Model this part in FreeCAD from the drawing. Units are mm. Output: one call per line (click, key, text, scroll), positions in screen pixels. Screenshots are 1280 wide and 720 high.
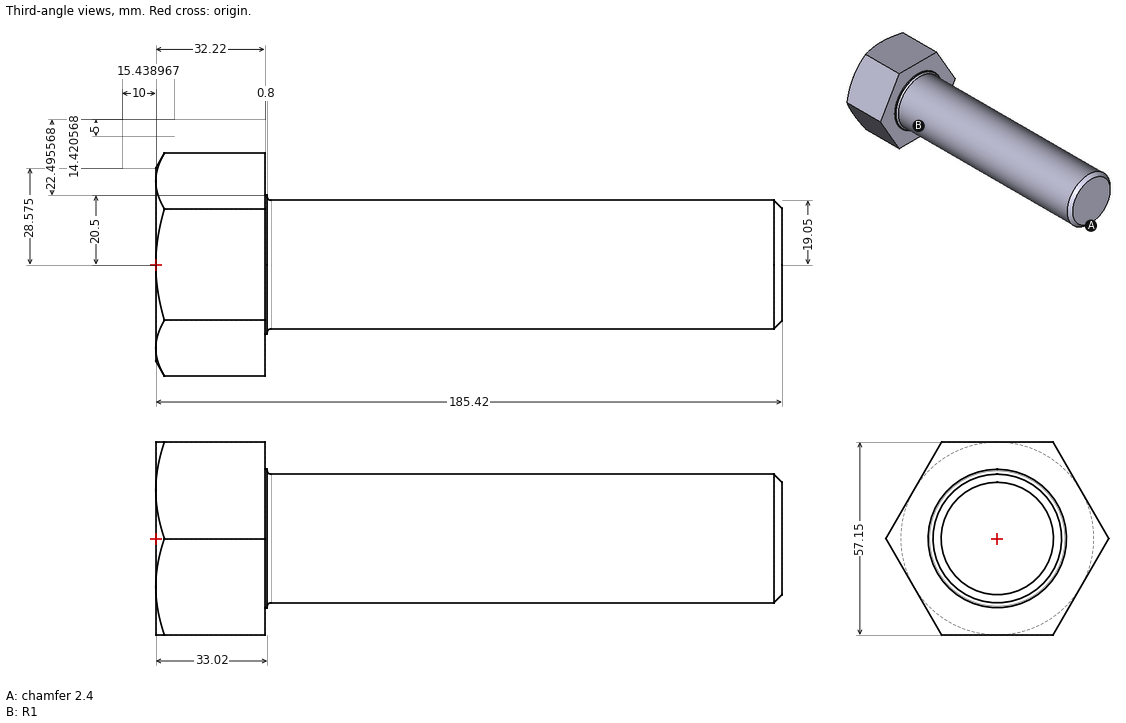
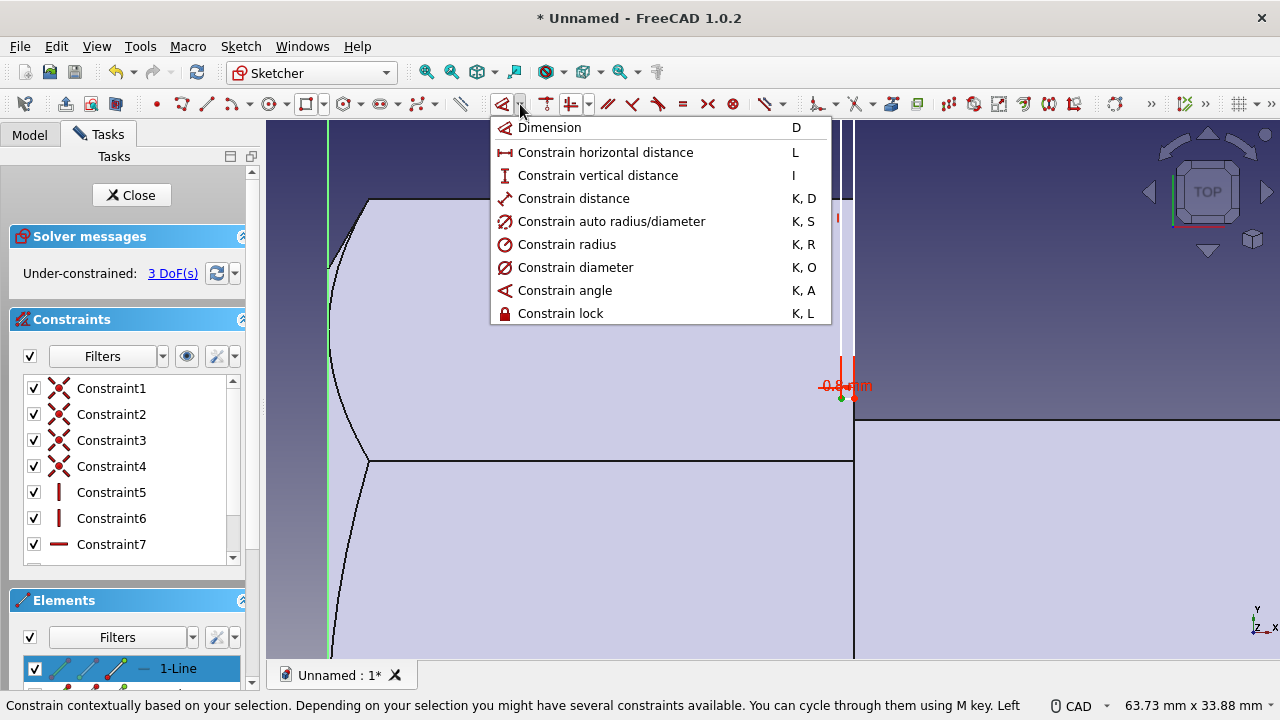
click(661, 176)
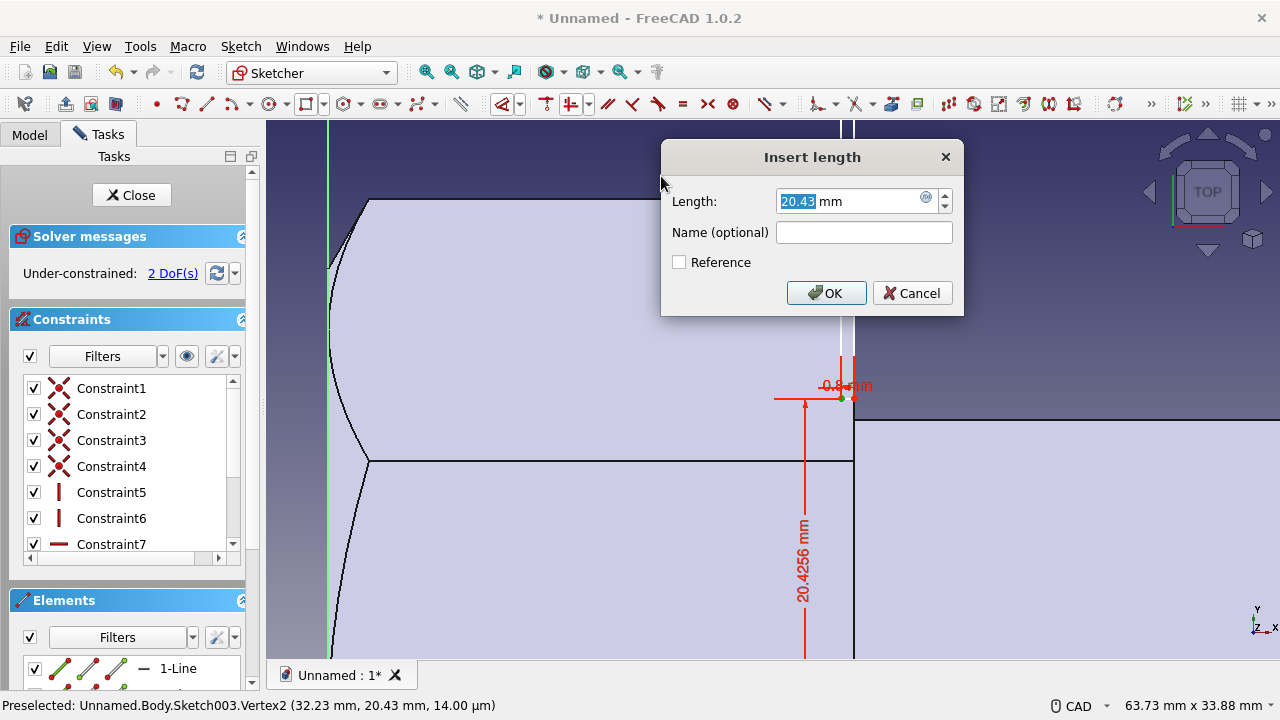
text(20.5)
key(Return)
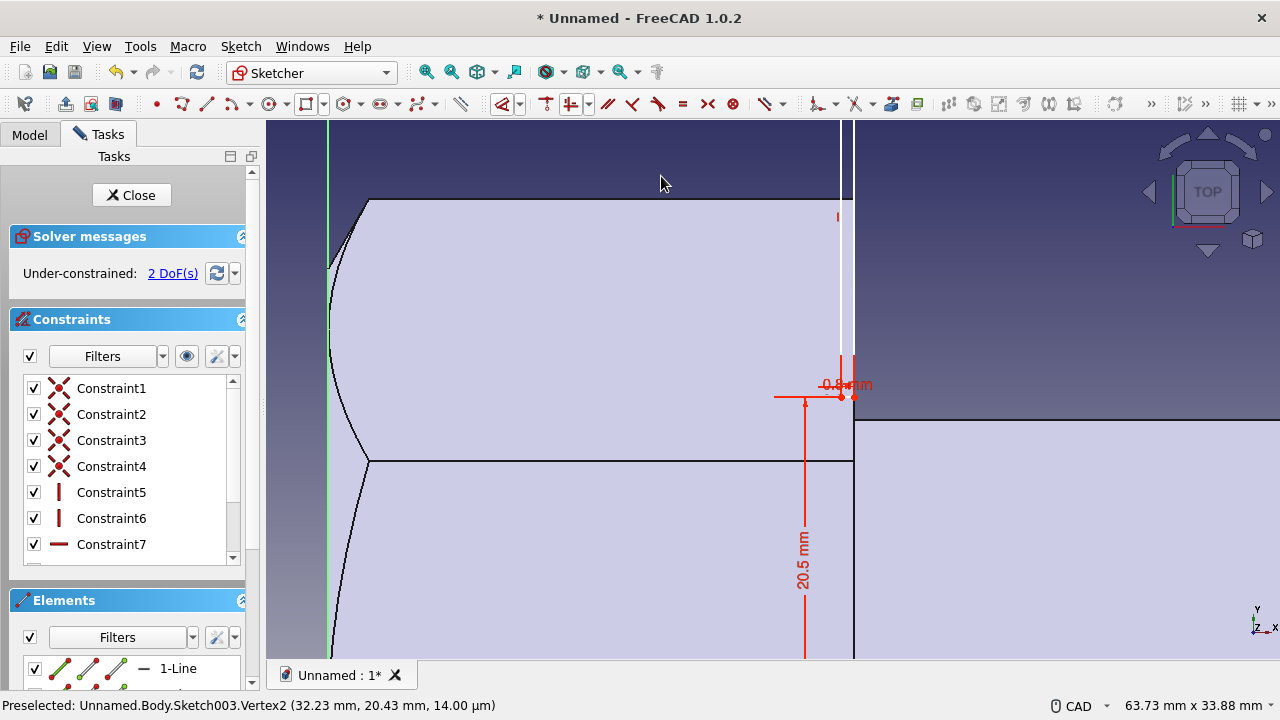
scroll(842, 399, down, 3)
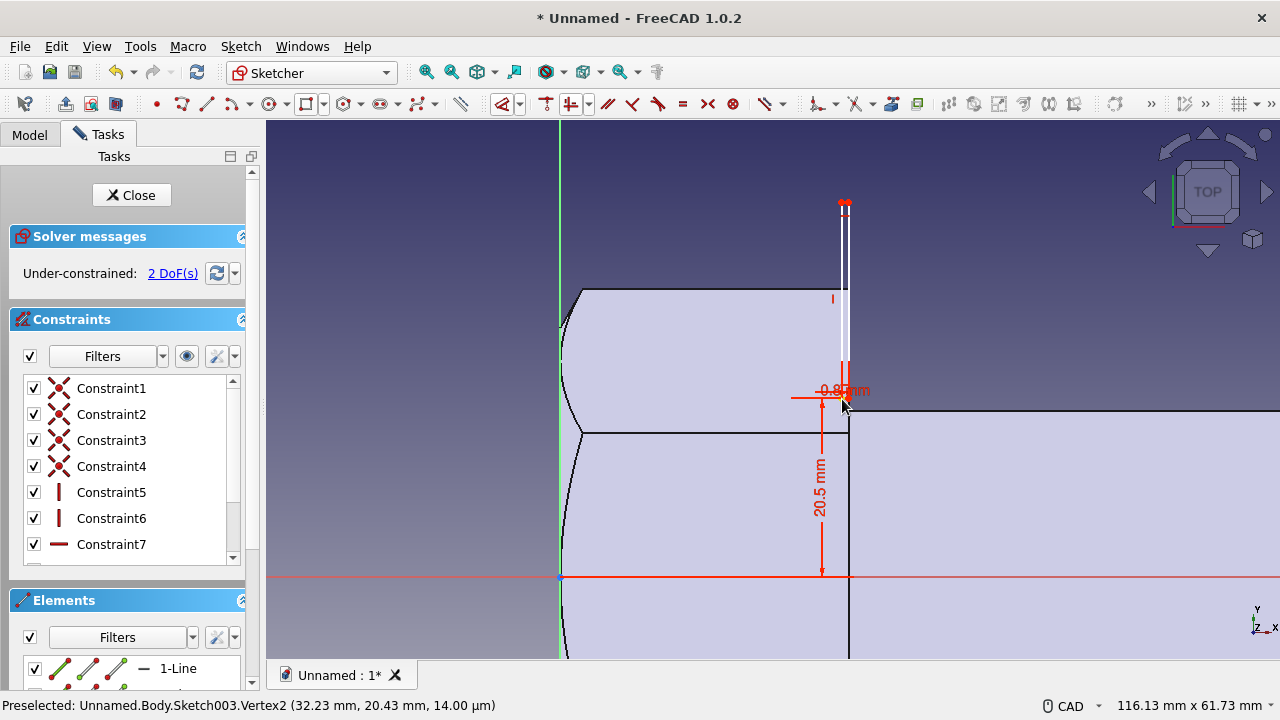
scroll(842, 202, up, 3)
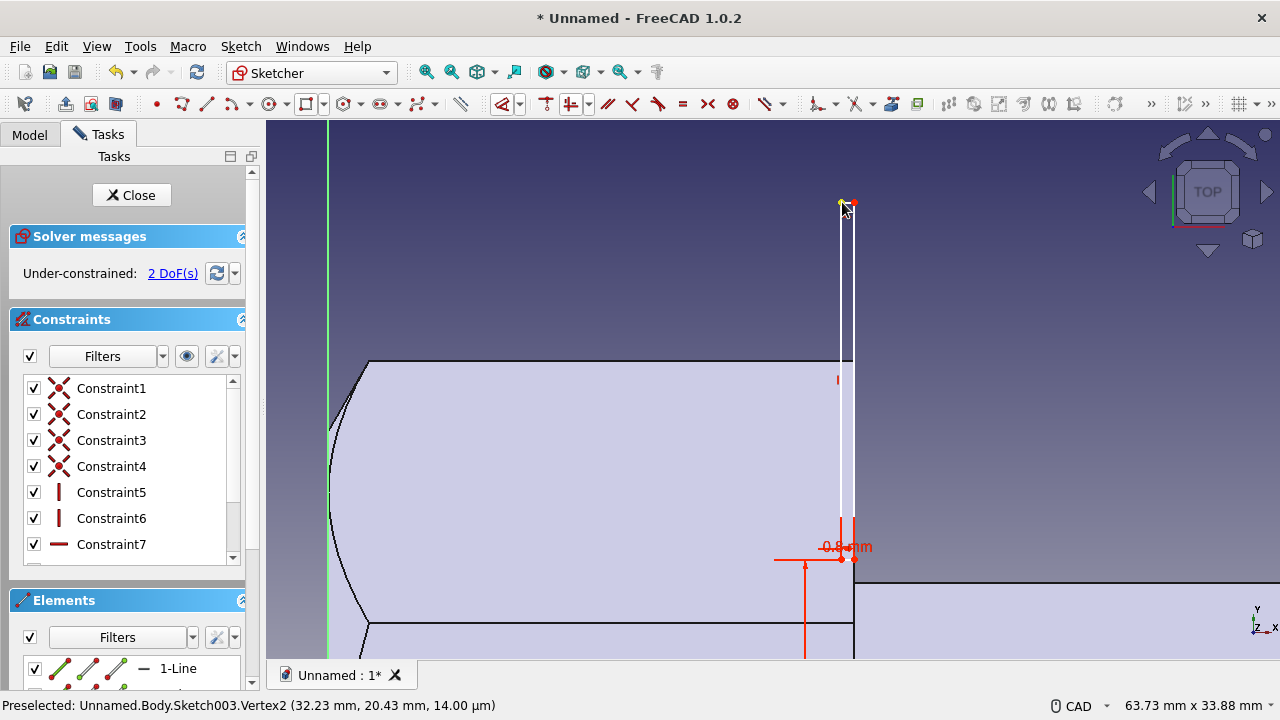
click(841, 203)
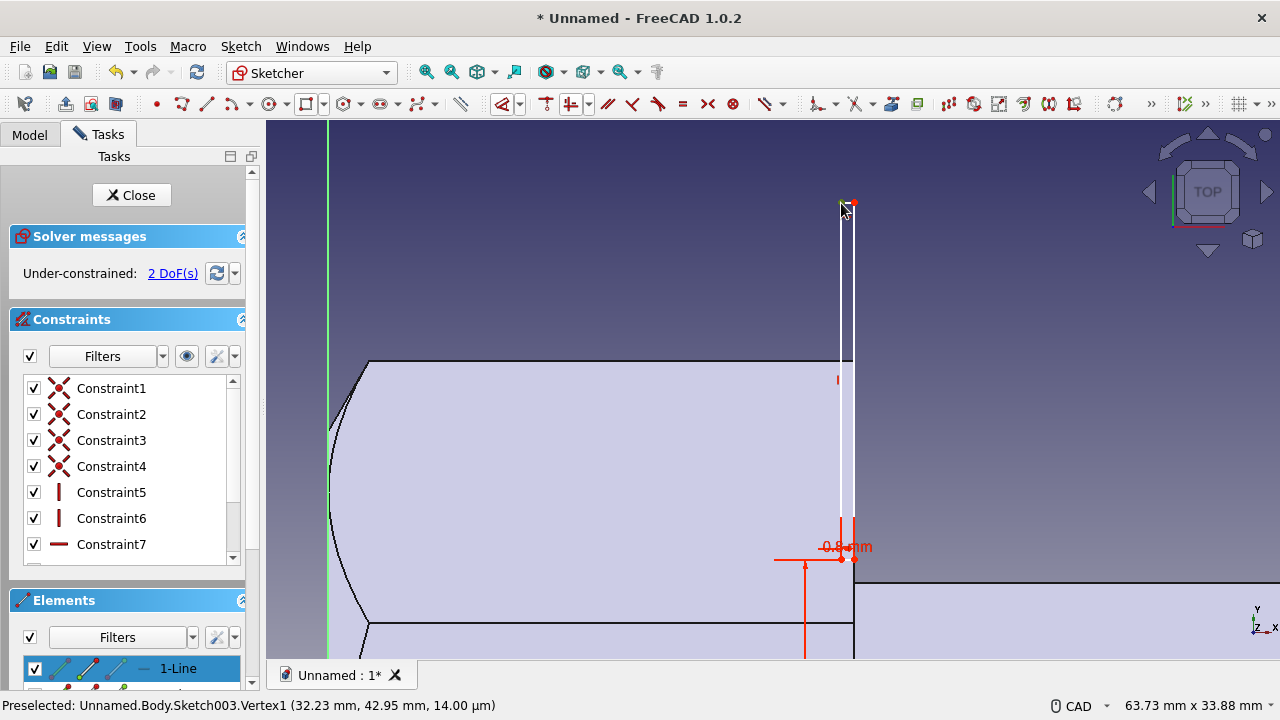
key(l)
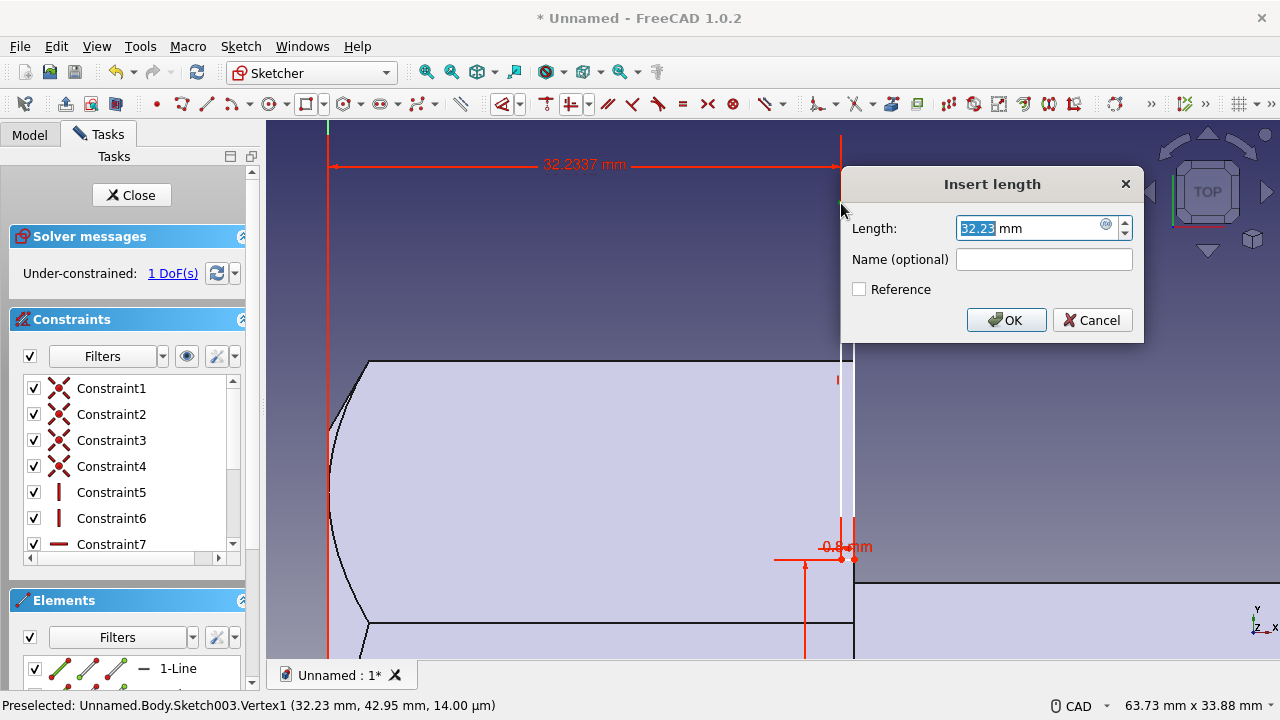
text(32.22)
key(Return)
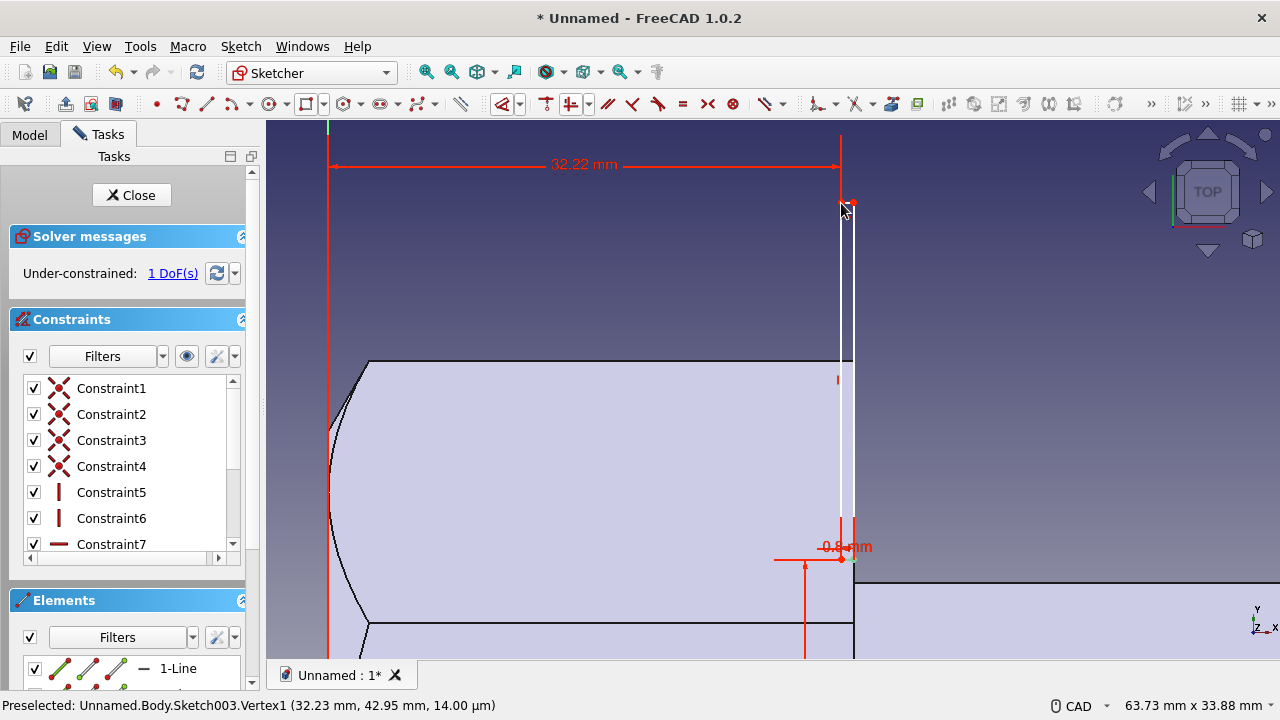
click(841, 310)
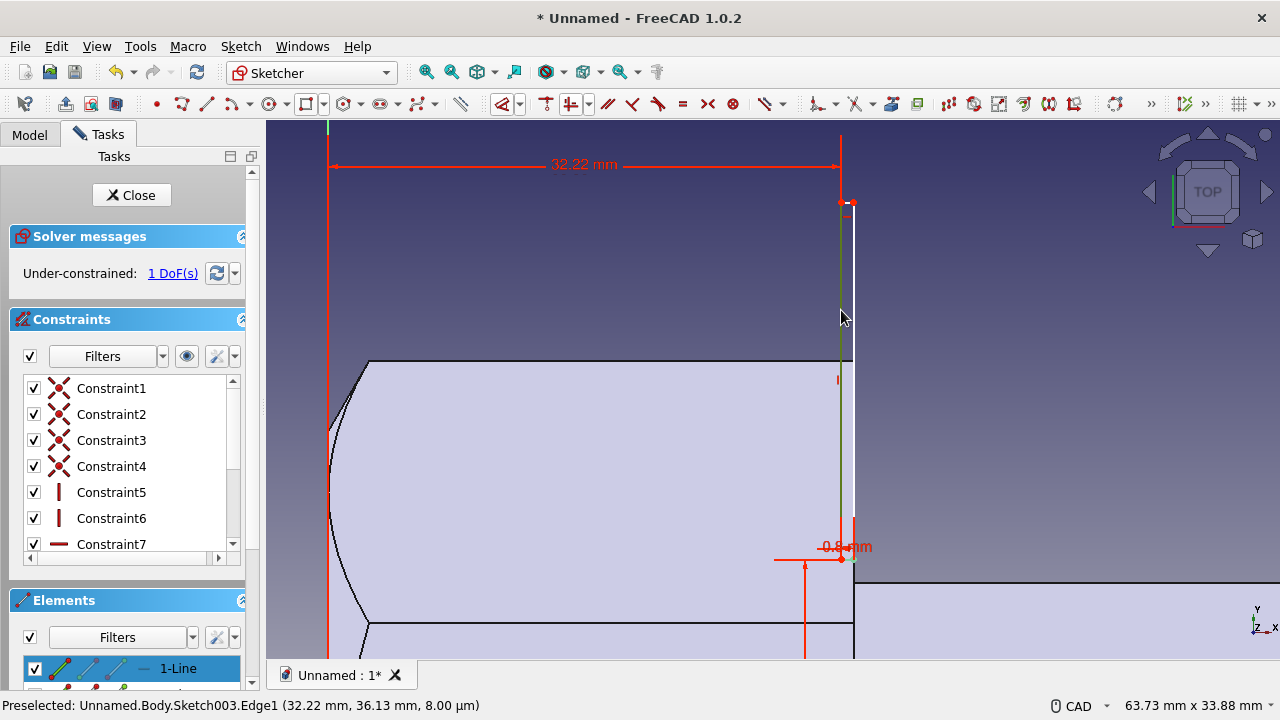
key(i)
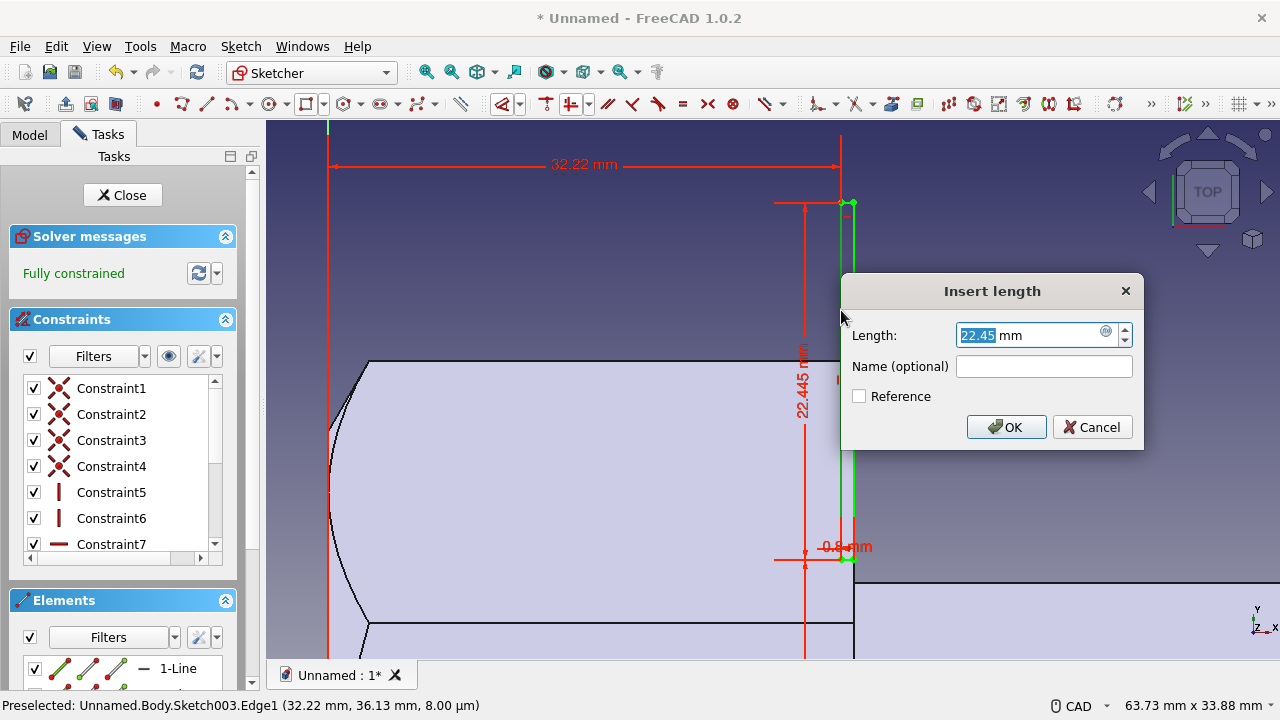
text(22.495568)
key(Return)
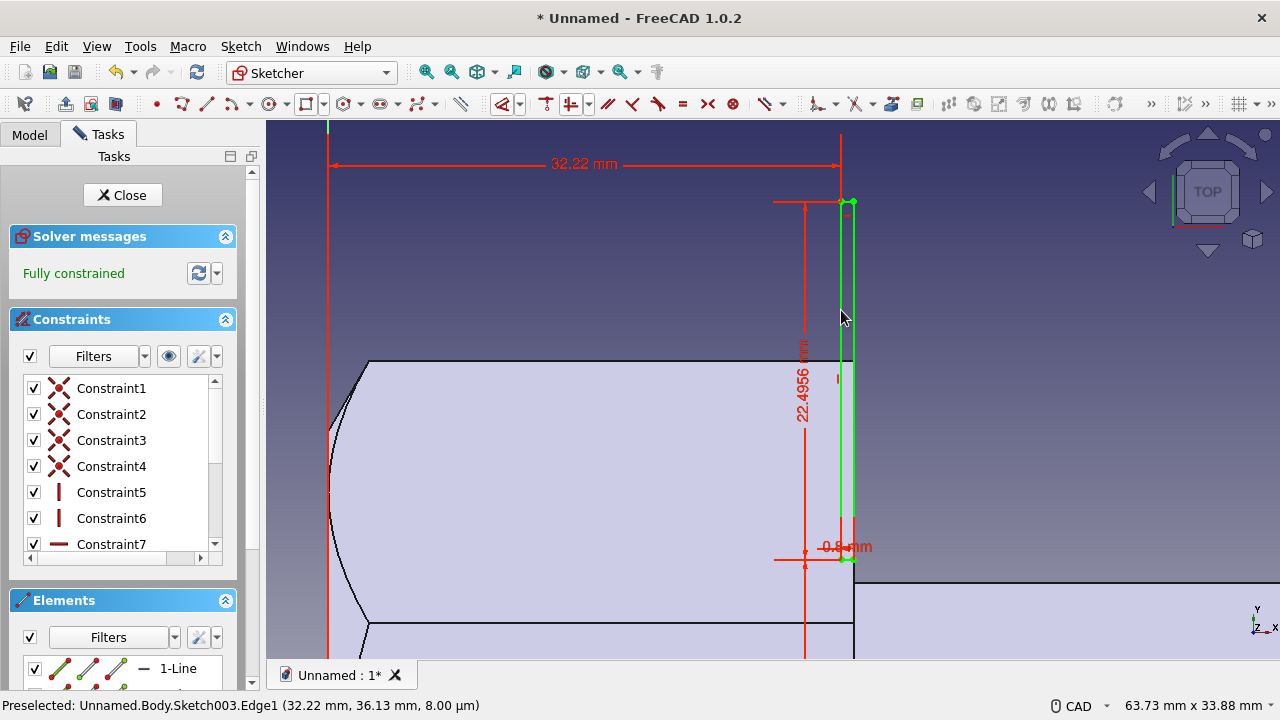
click(123, 195)